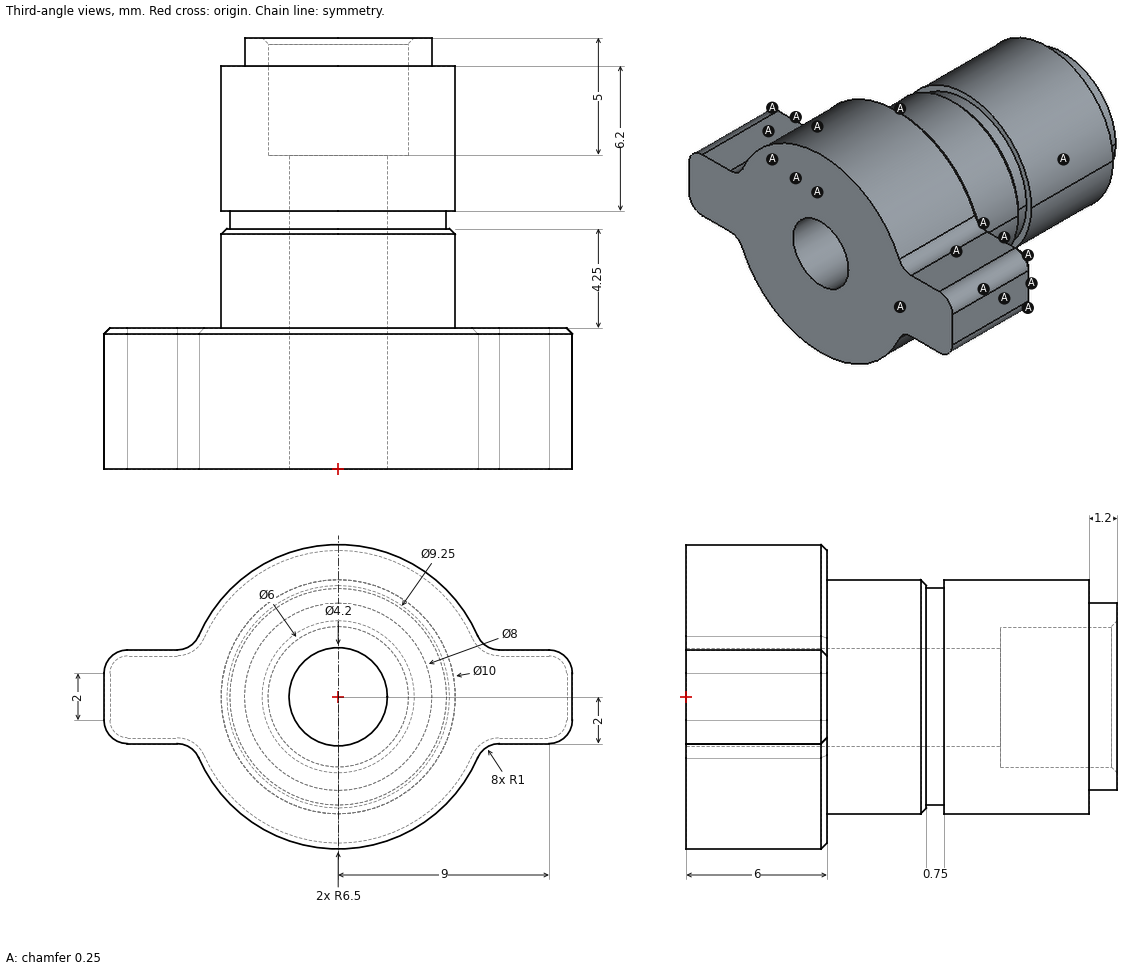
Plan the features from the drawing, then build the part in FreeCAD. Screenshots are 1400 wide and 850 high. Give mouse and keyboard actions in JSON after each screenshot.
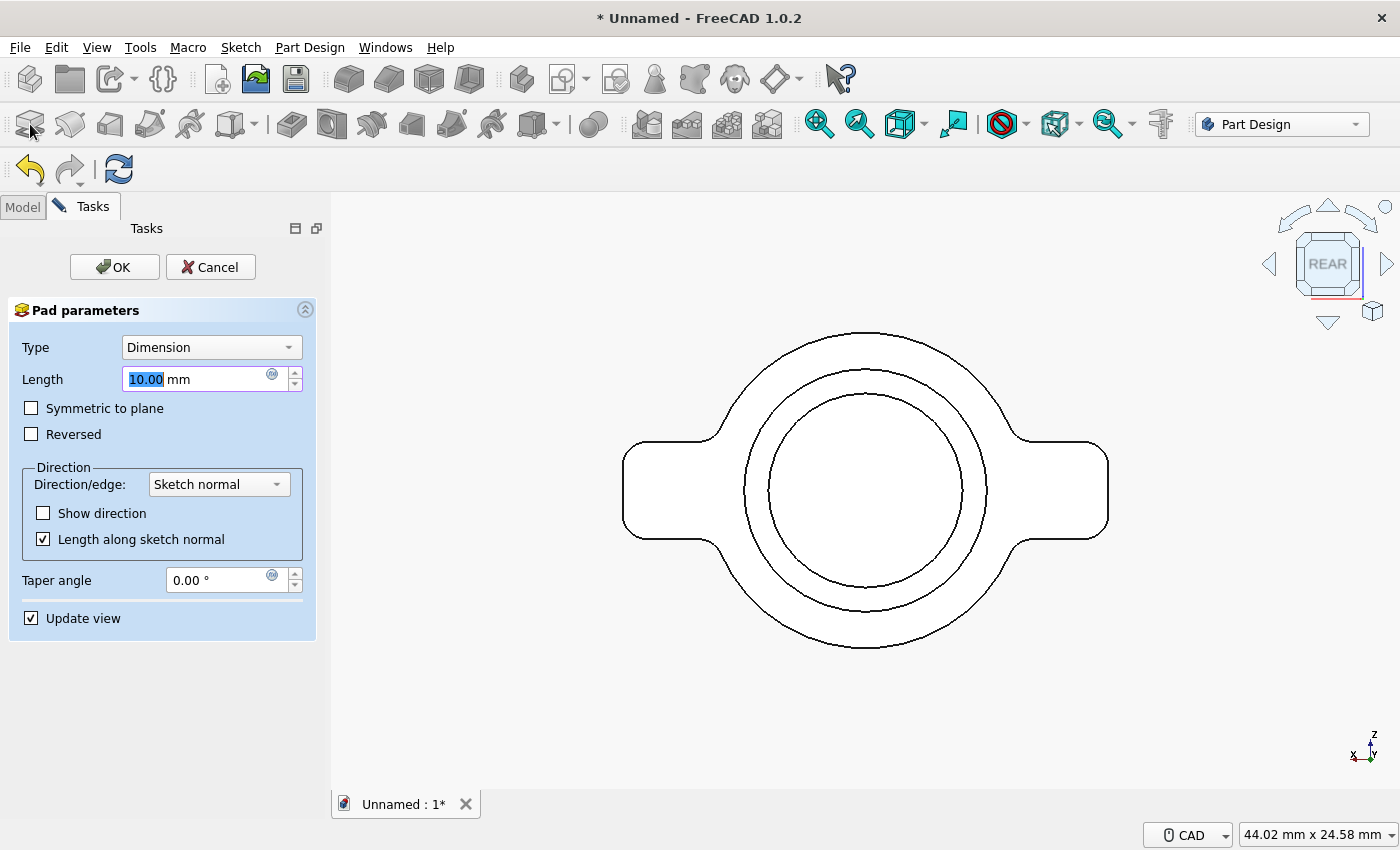
{"action": "type", "text": "1.2"}
{"action": "key", "text": "Tab"}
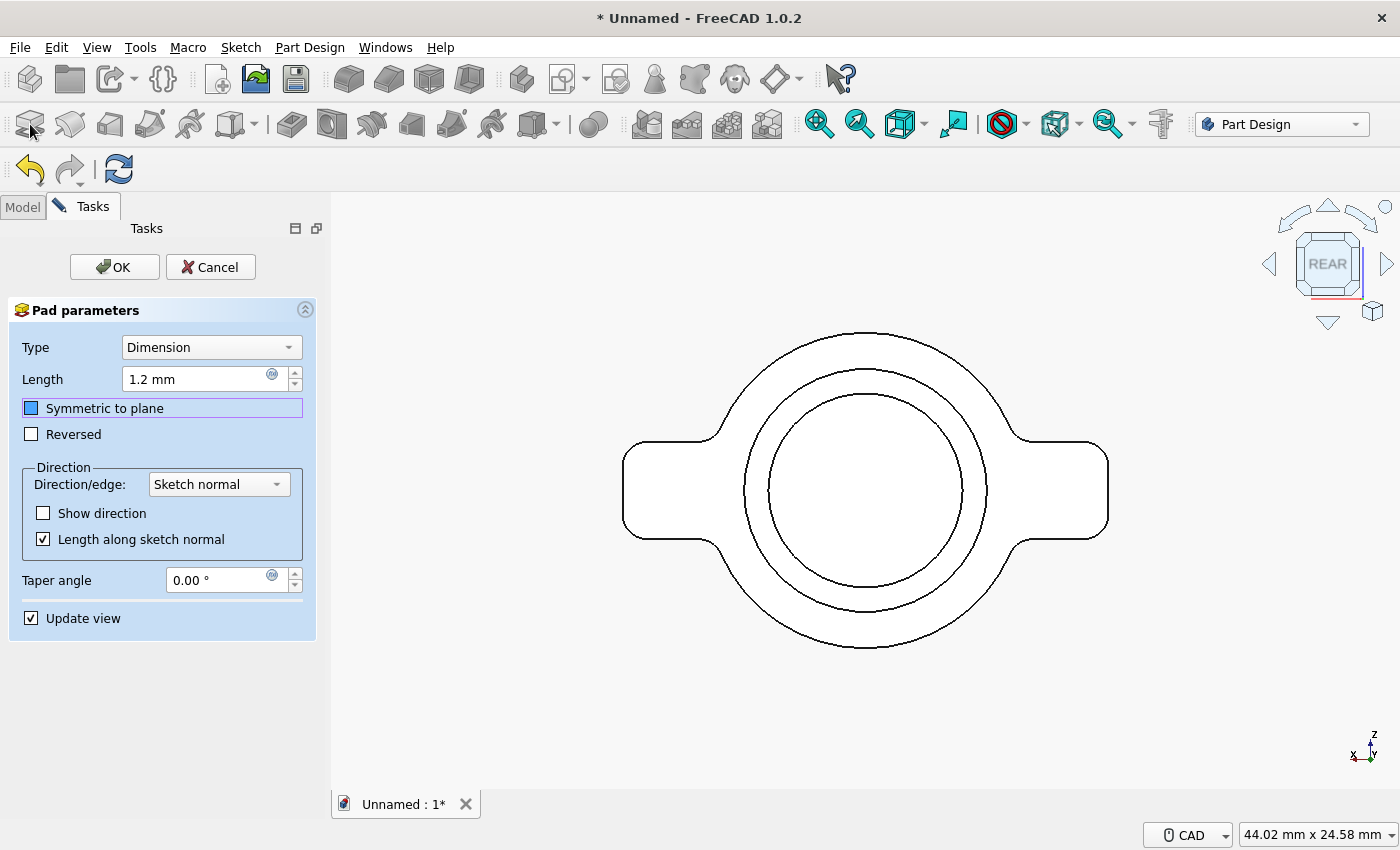
{"action": "left_click", "coordinate": [115, 267]}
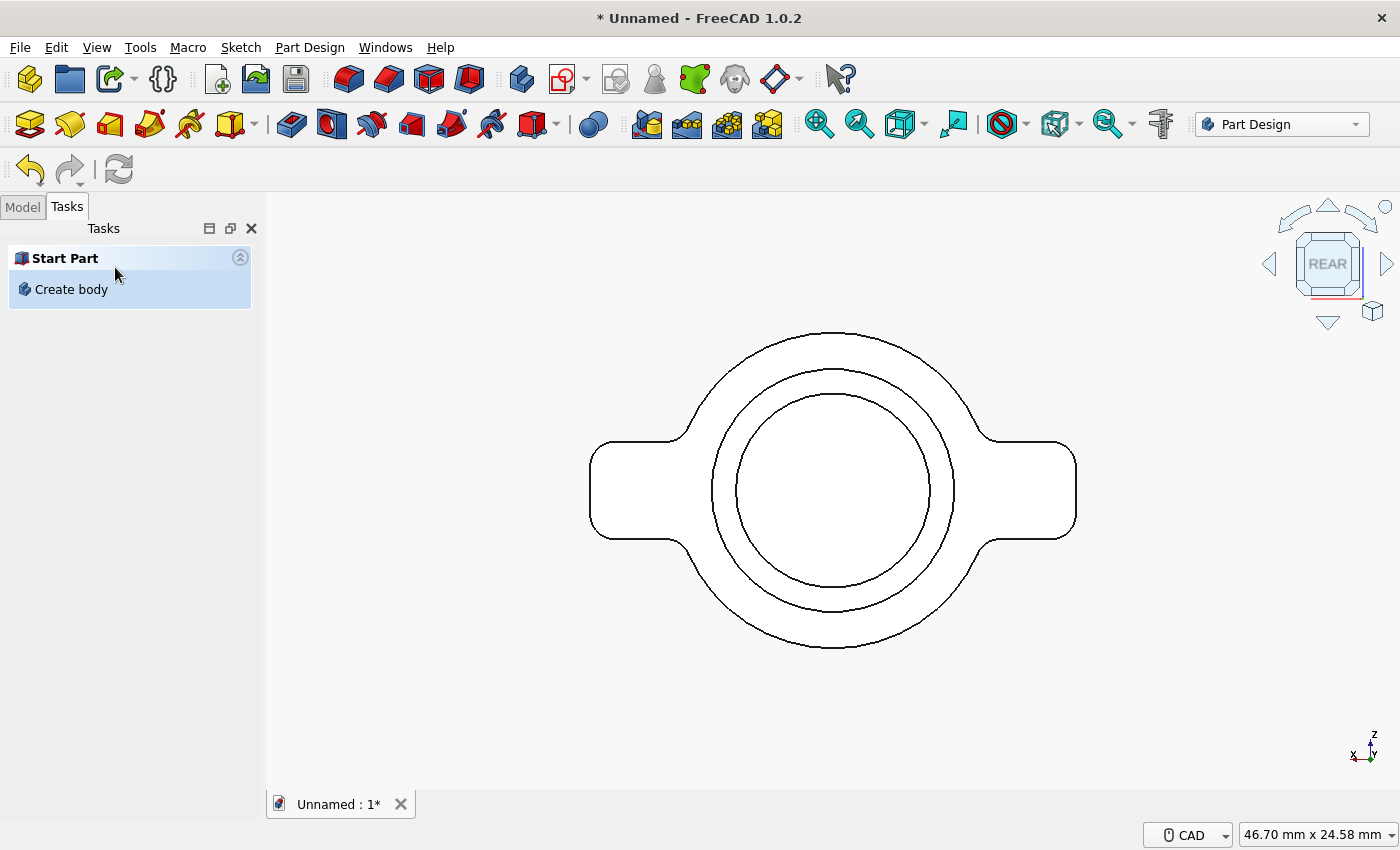
{"action": "left_click", "coordinate": [833, 490]}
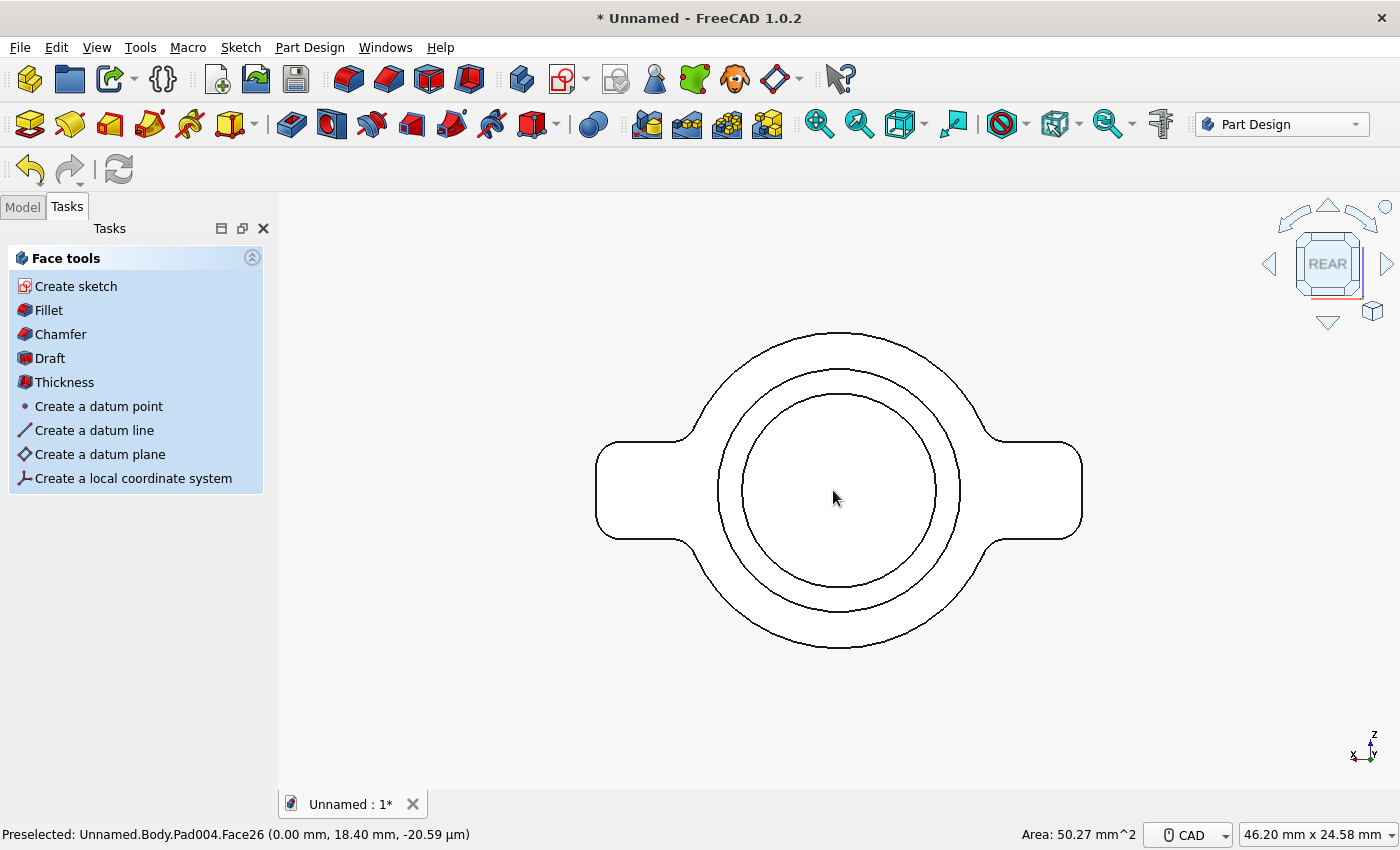
{"action": "left_click", "coordinate": [562, 80]}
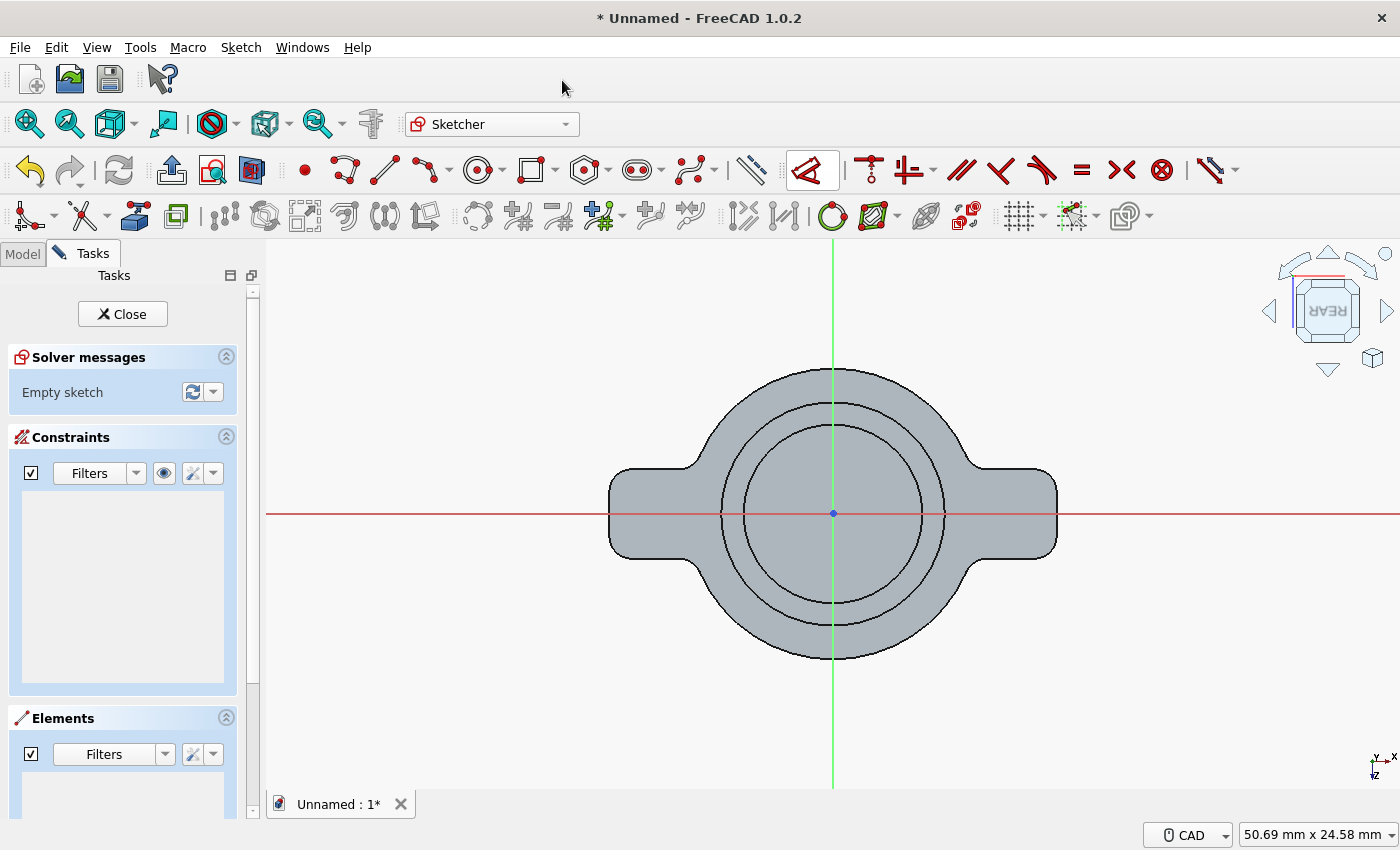
{"action": "scroll", "coordinate": [873, 514], "scroll_direction": "up", "scroll_amount": 5}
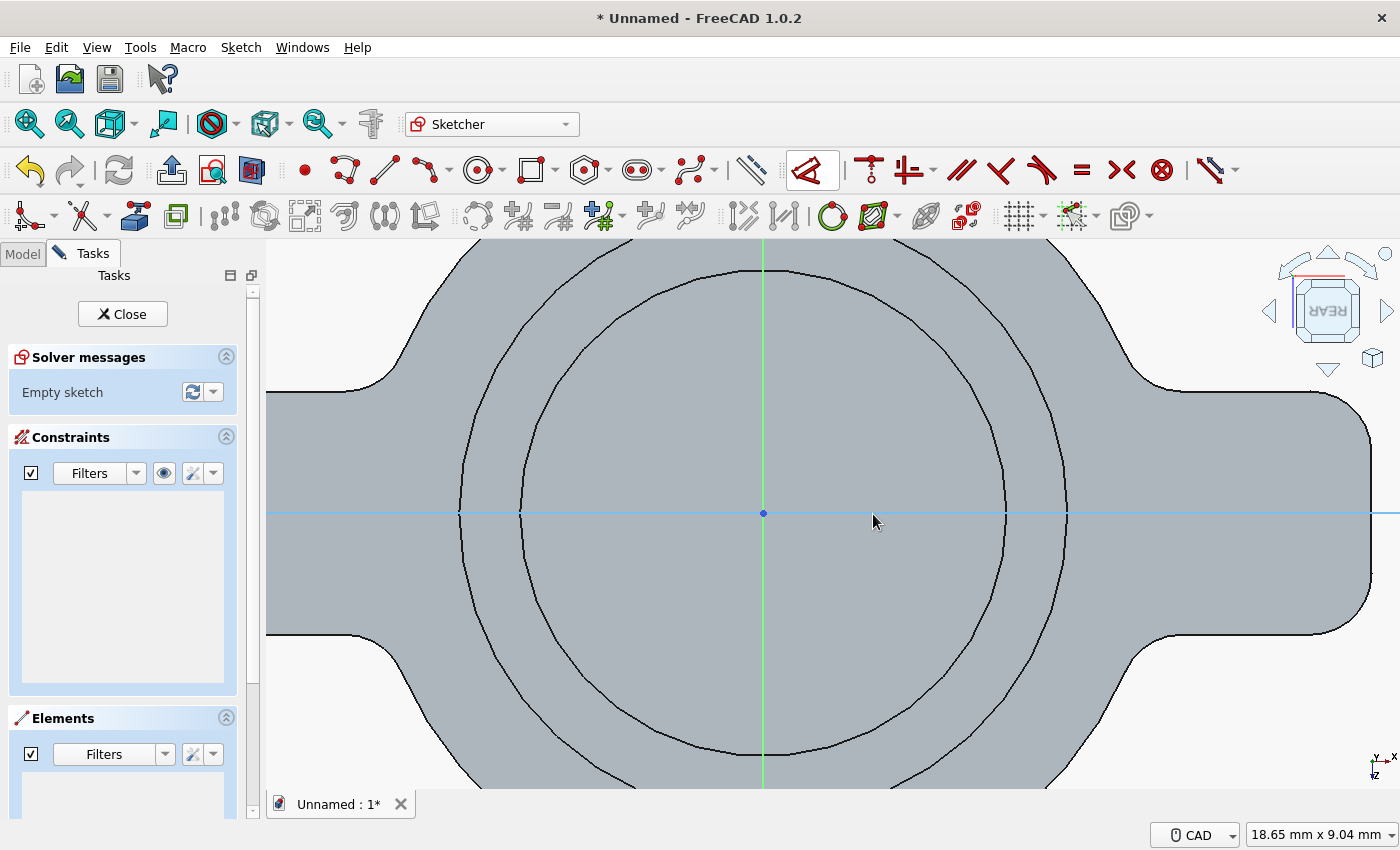
{"action": "left_click", "coordinate": [478, 170]}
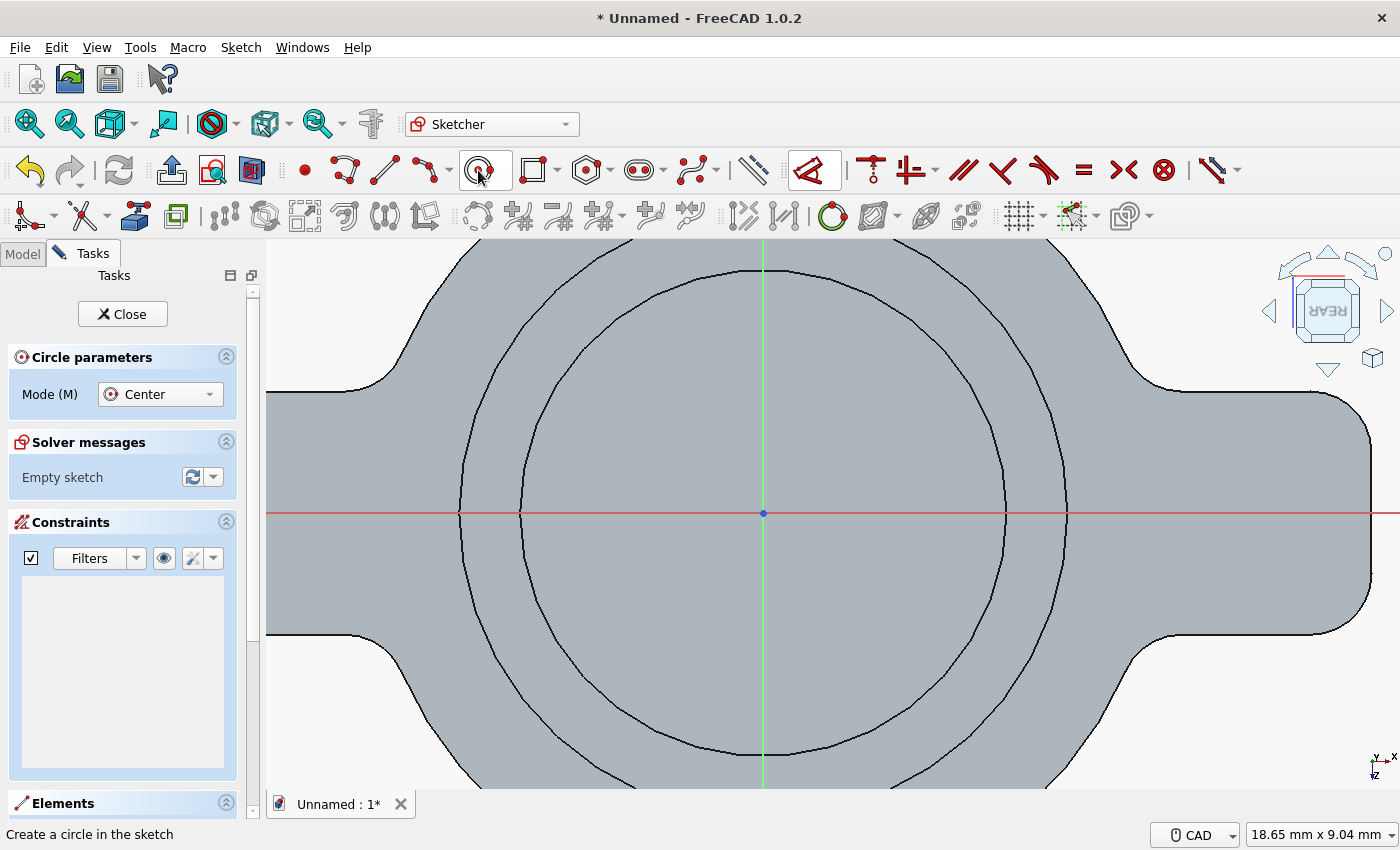
{"action": "left_click", "coordinate": [763, 513]}
{"action": "mouse_move", "coordinate": [892, 384]}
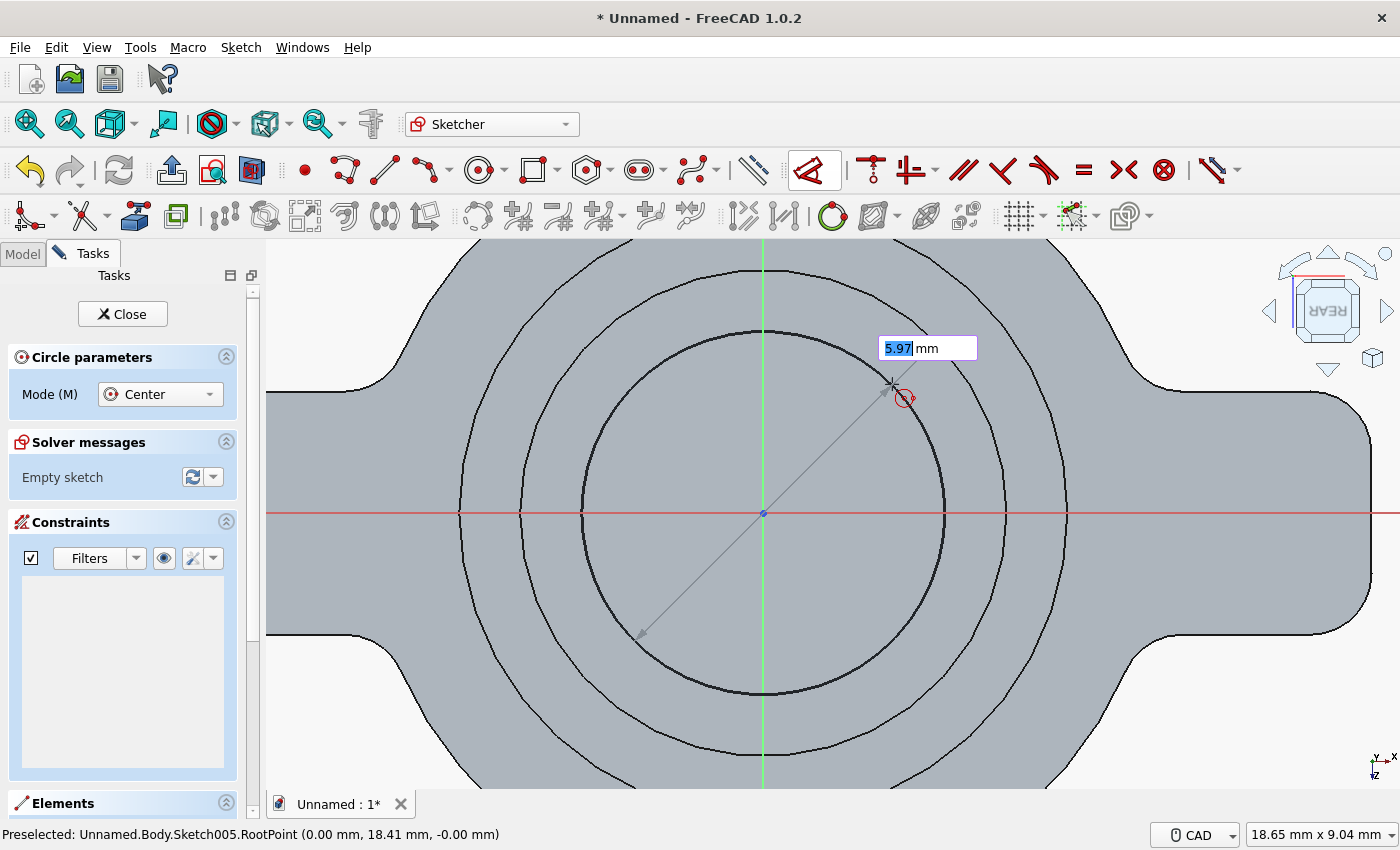
{"action": "type", "text": "6"}
{"action": "key", "text": "Return"}
{"action": "key", "text": "Escape"}